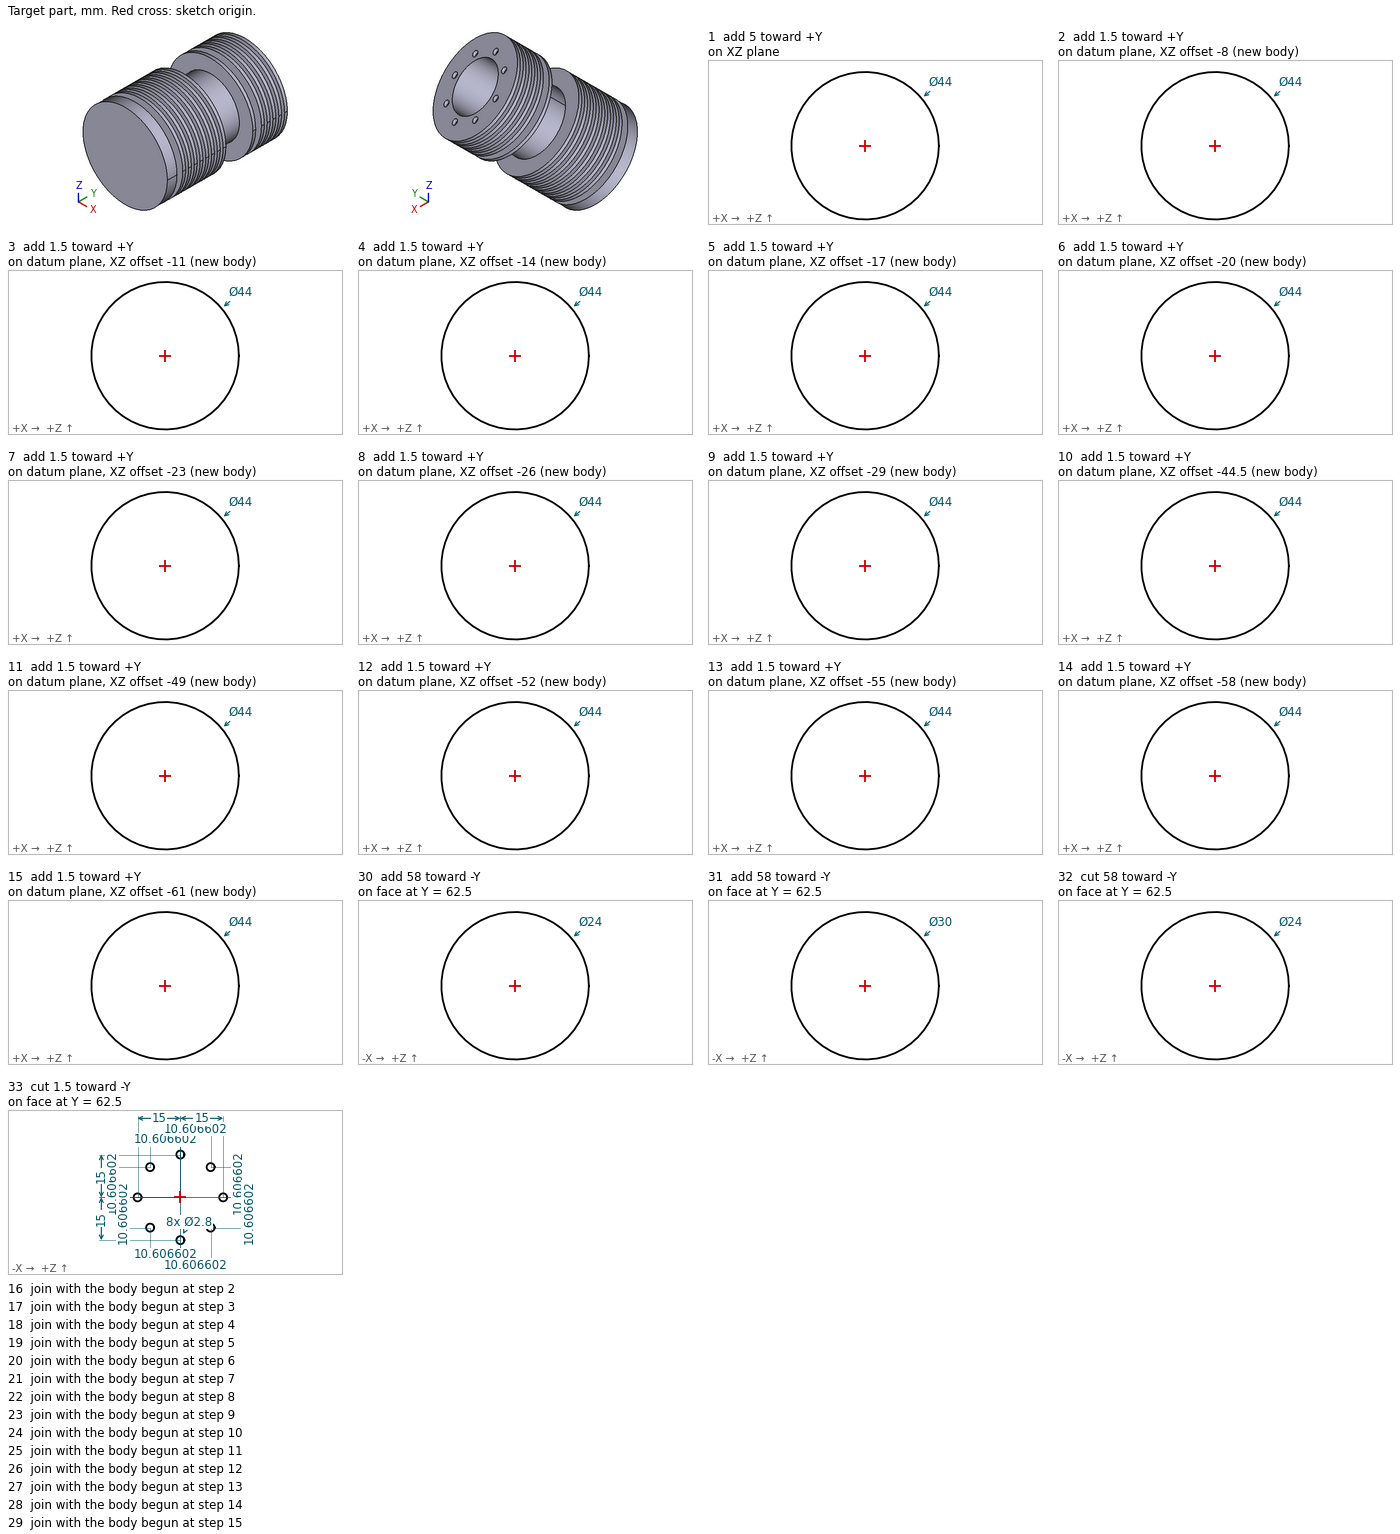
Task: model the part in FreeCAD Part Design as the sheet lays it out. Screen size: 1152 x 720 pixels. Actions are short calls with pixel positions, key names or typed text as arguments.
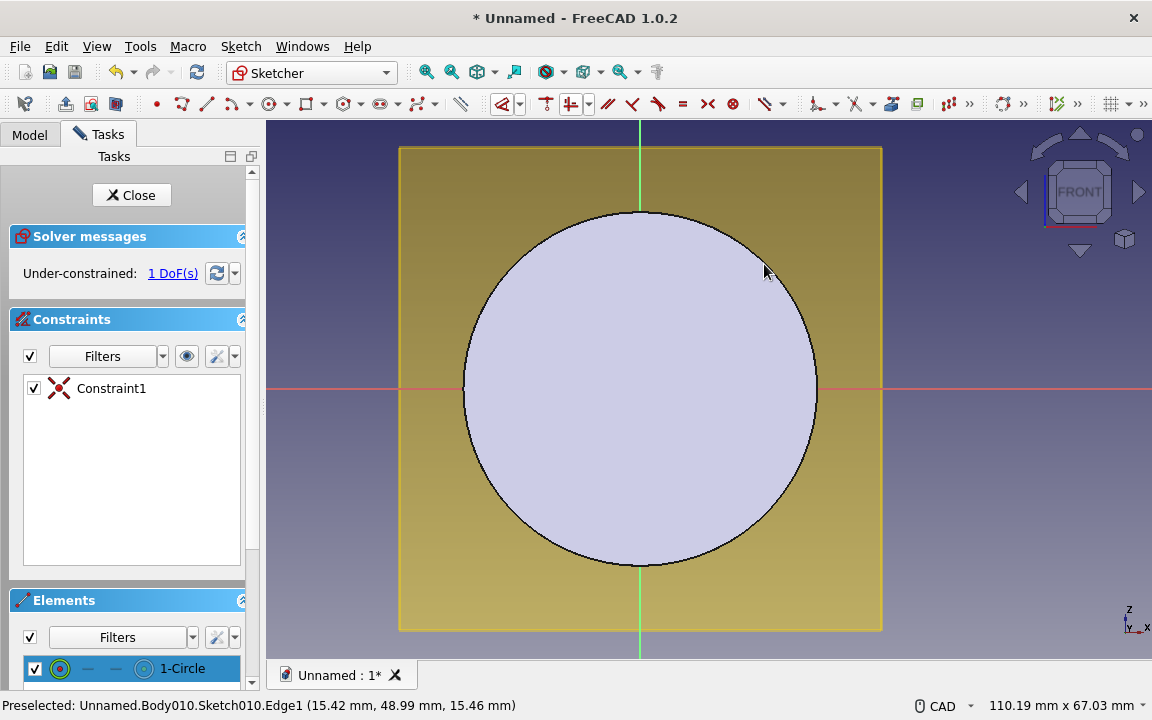
key(k)
key(o)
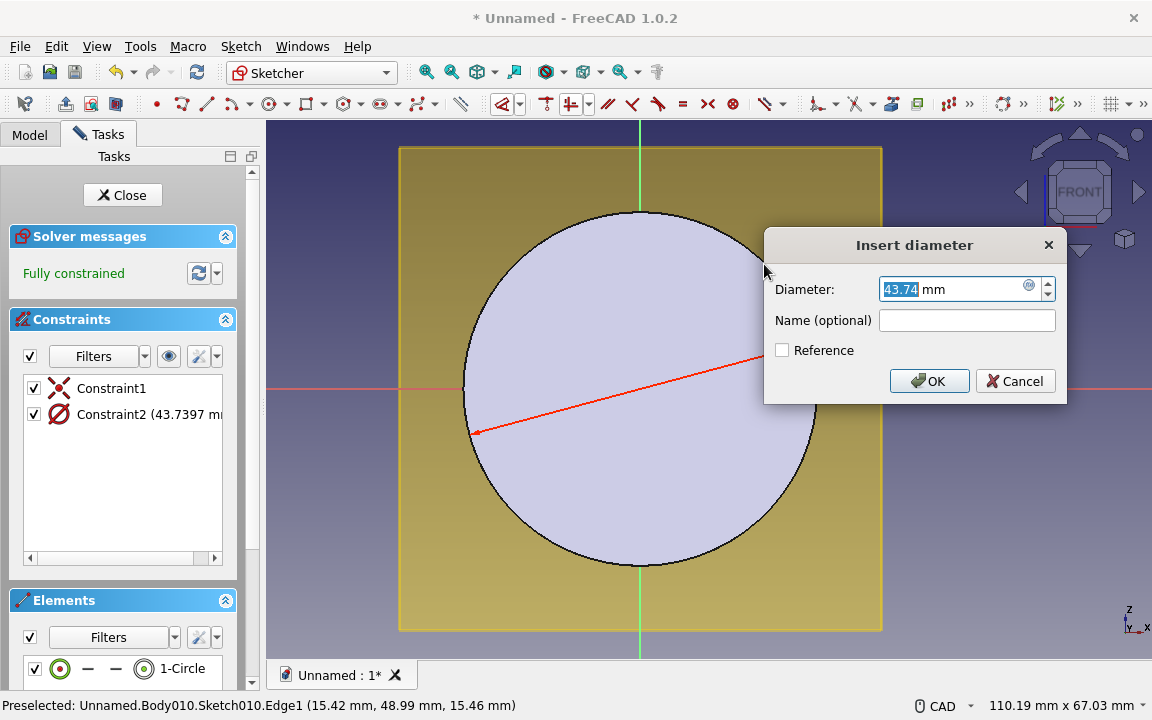
text(44)
key(Return)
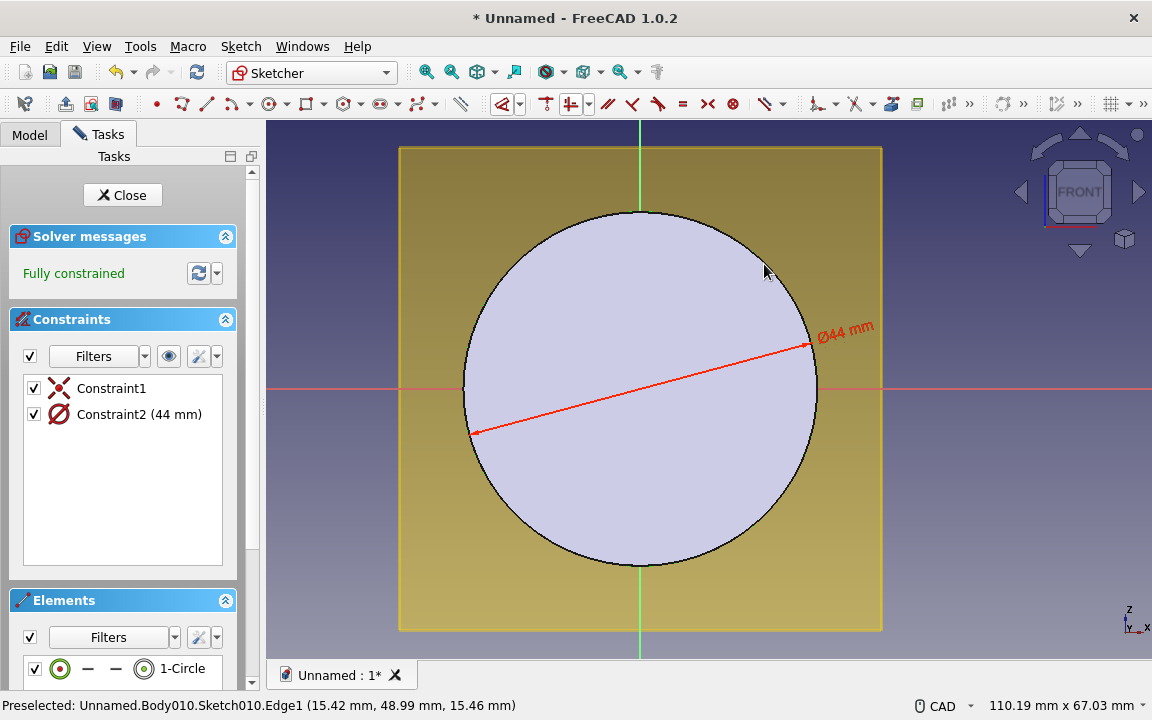
click(123, 195)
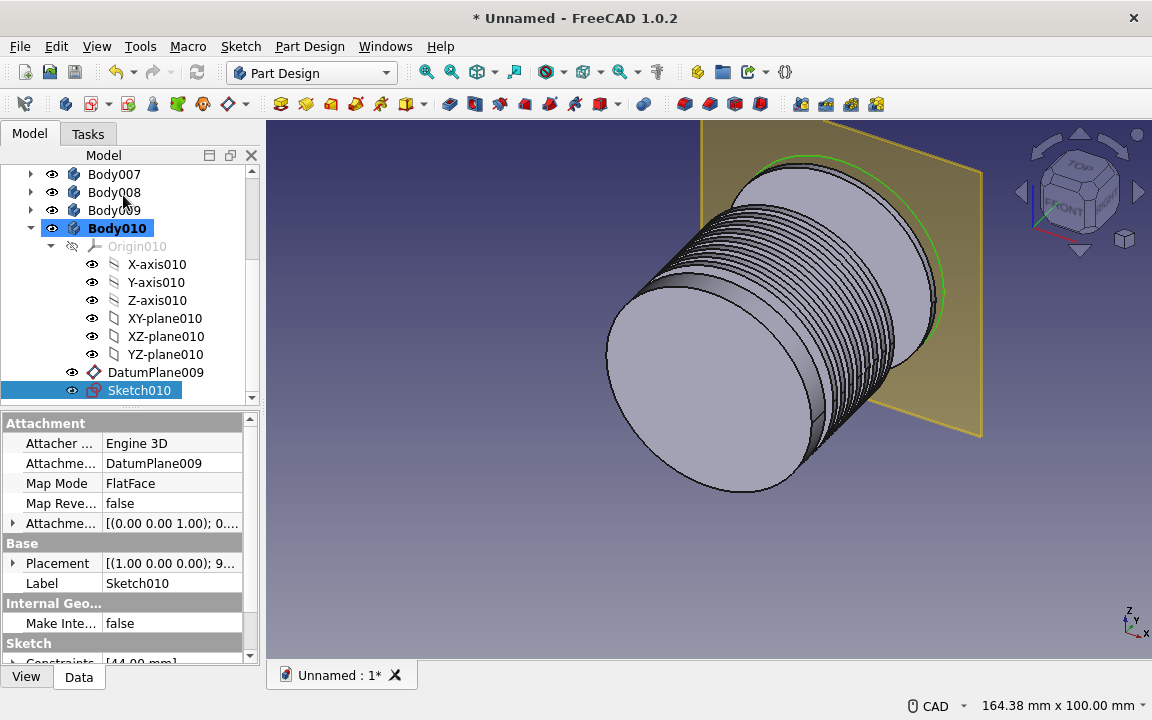
click(281, 104)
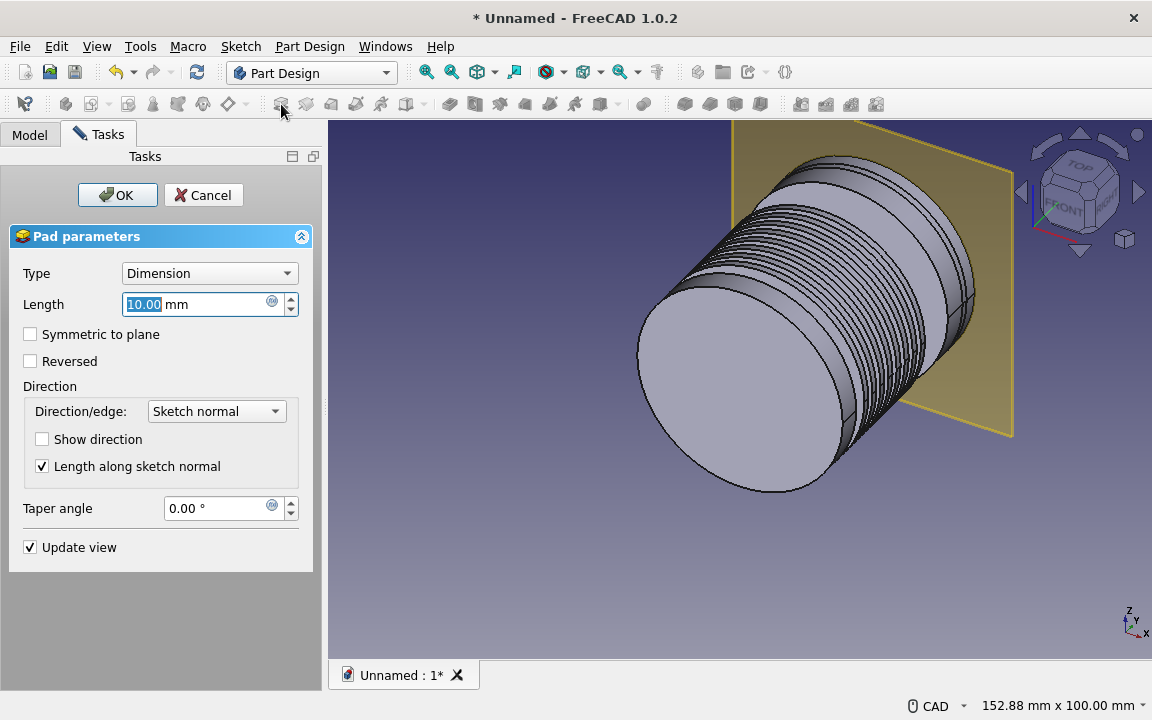
text(1.5)
key(Tab)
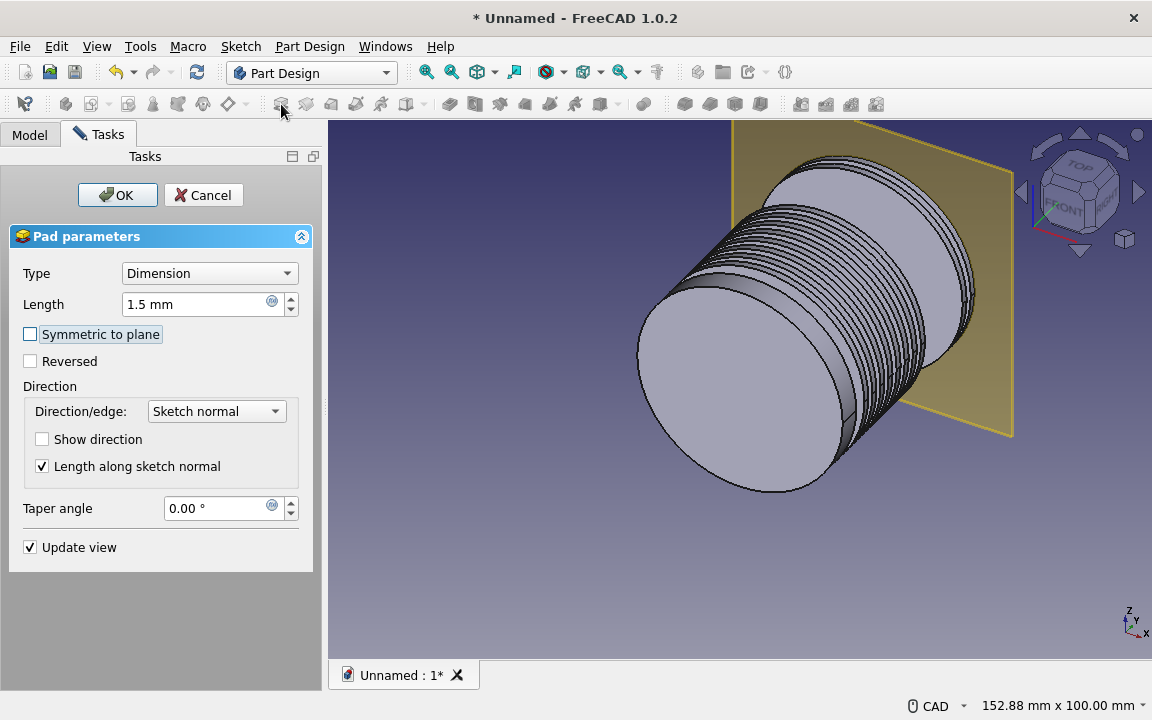
click(31, 361)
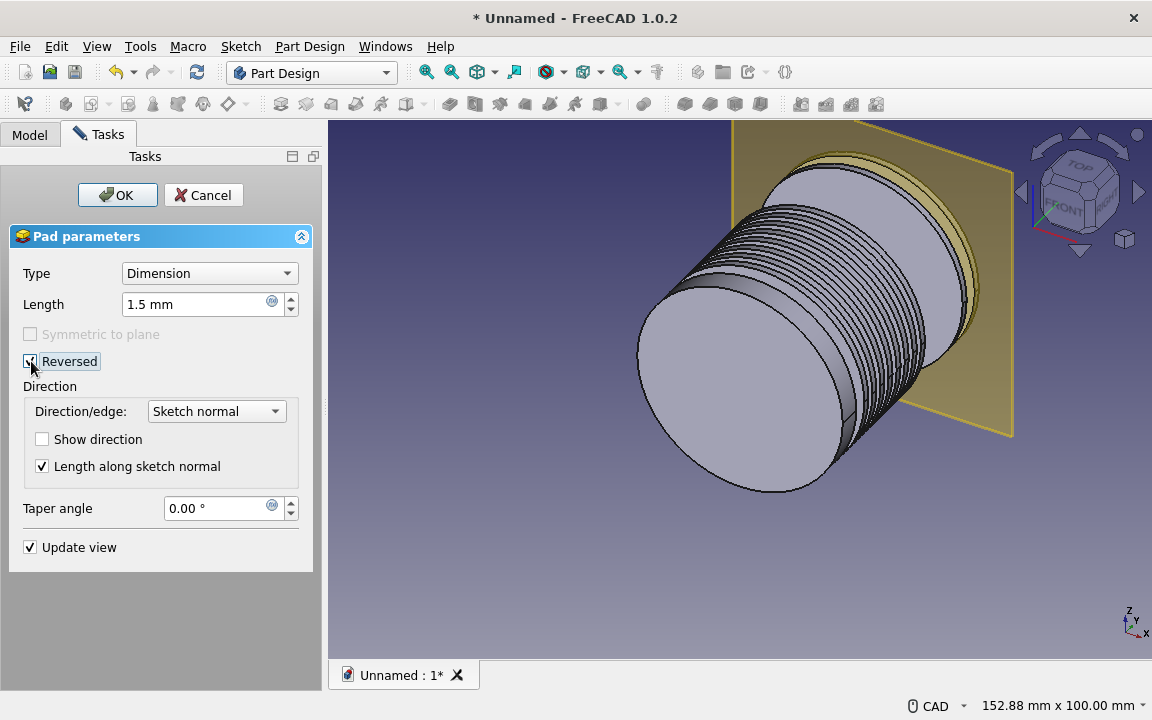
click(118, 195)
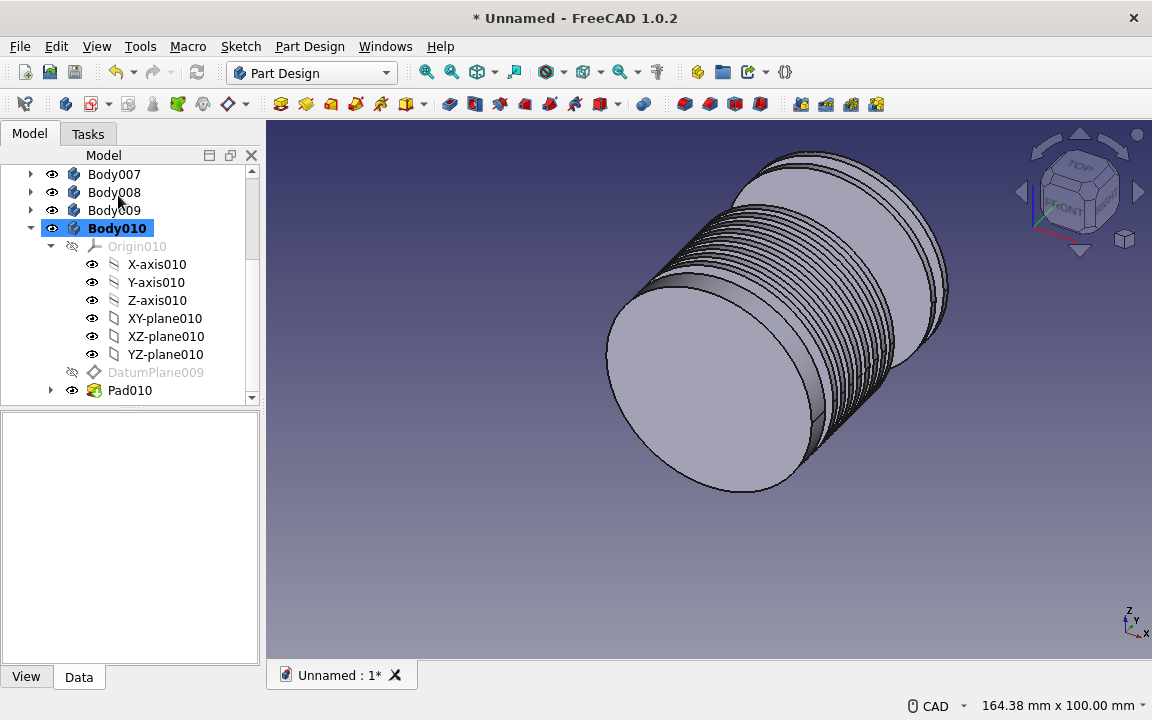
click(66, 104)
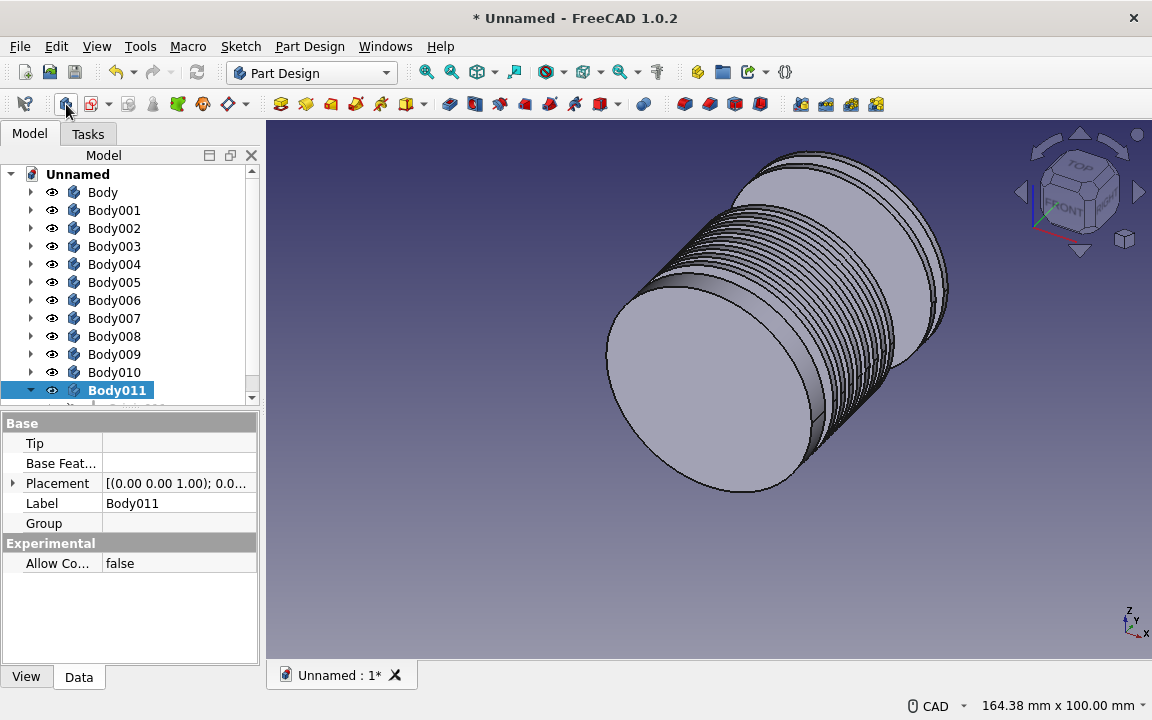
scroll(101, 278, down, 3)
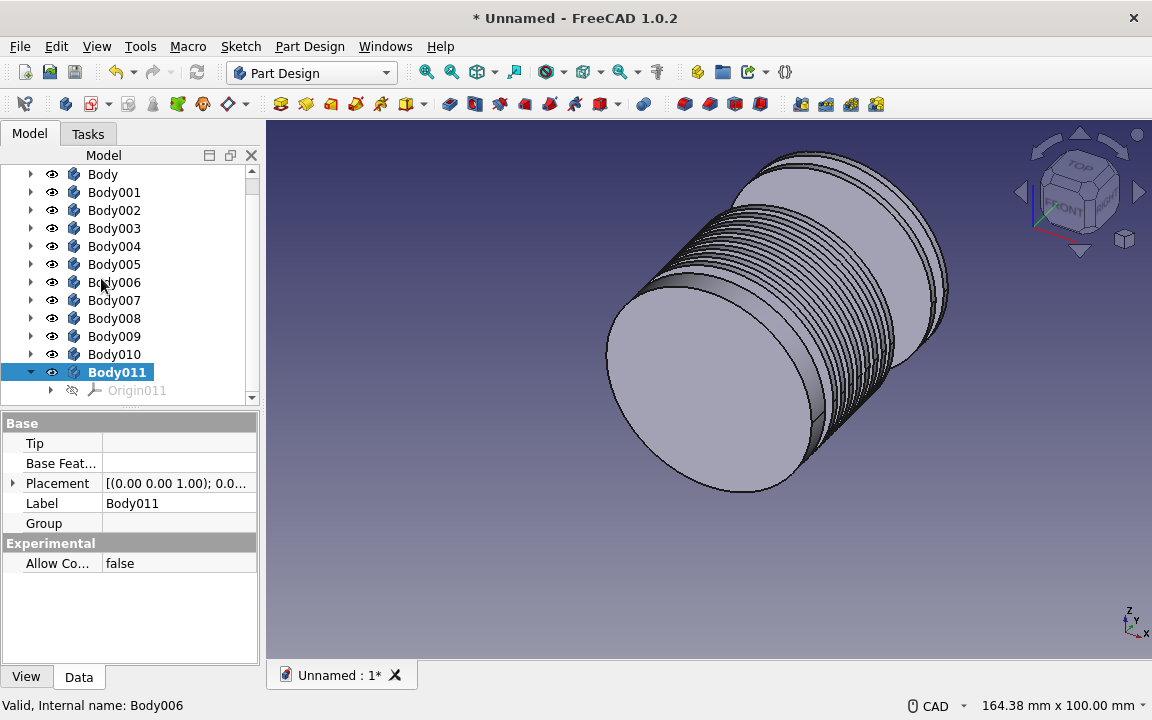
click(51, 390)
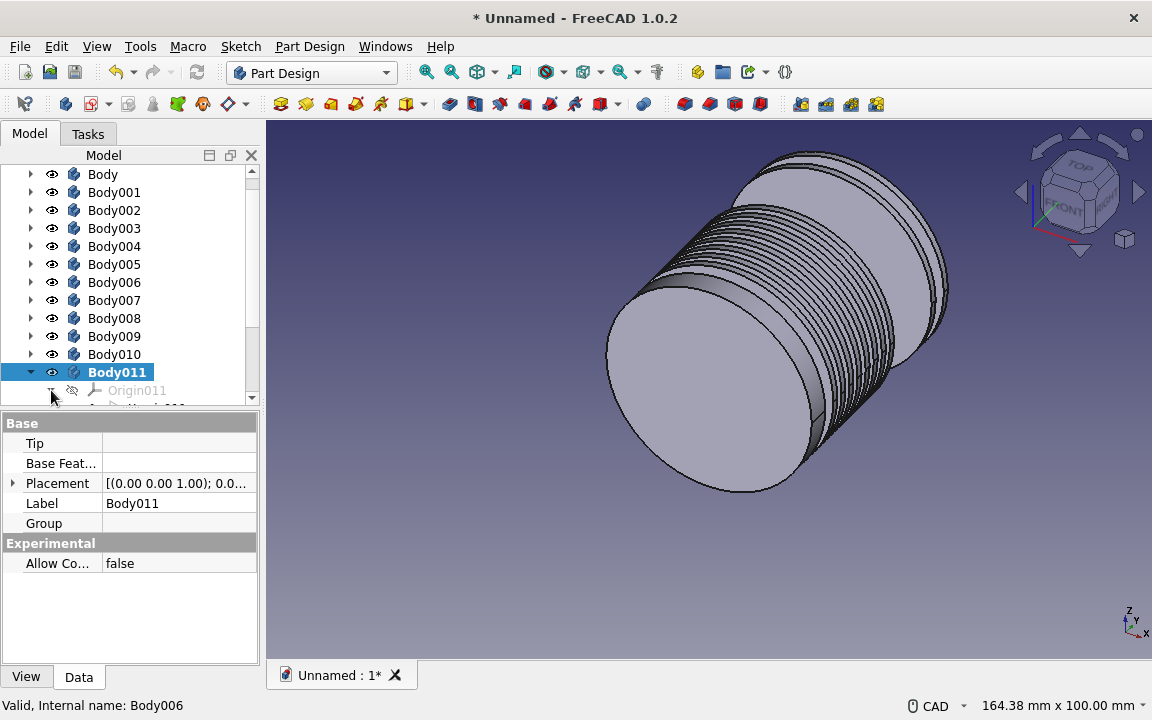
scroll(121, 278, down, 3)